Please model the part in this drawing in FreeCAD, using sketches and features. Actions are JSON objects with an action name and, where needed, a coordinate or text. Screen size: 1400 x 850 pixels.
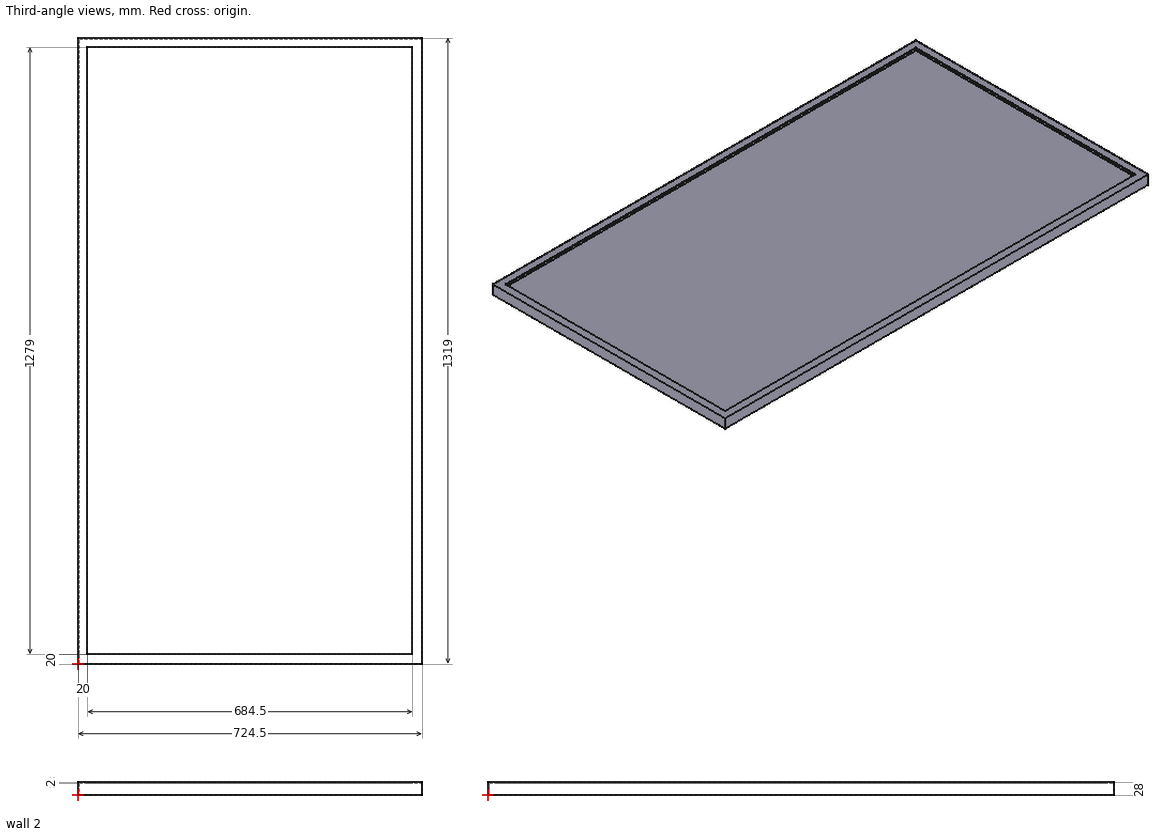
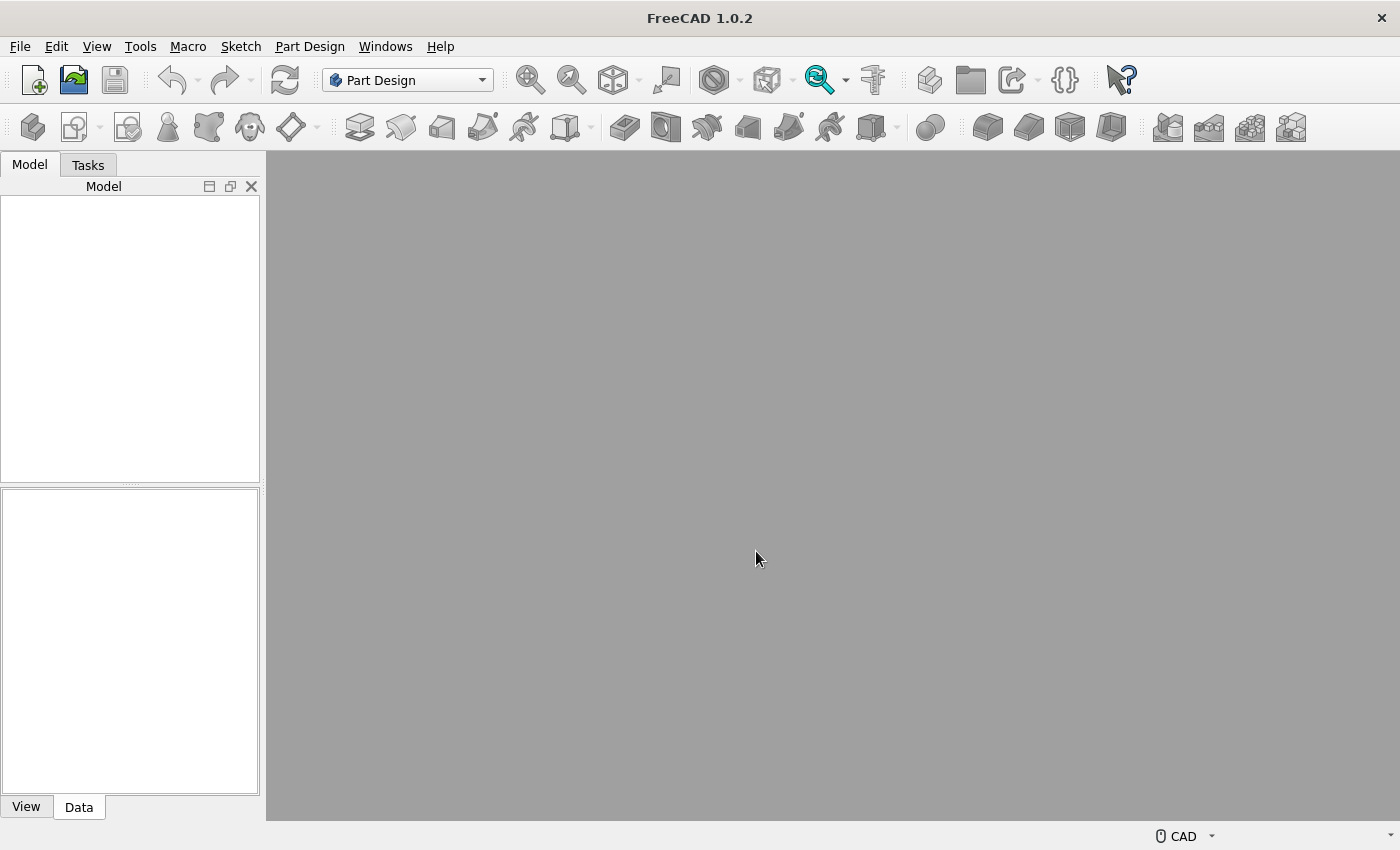
{"action": "left_click", "coordinate": [33, 80]}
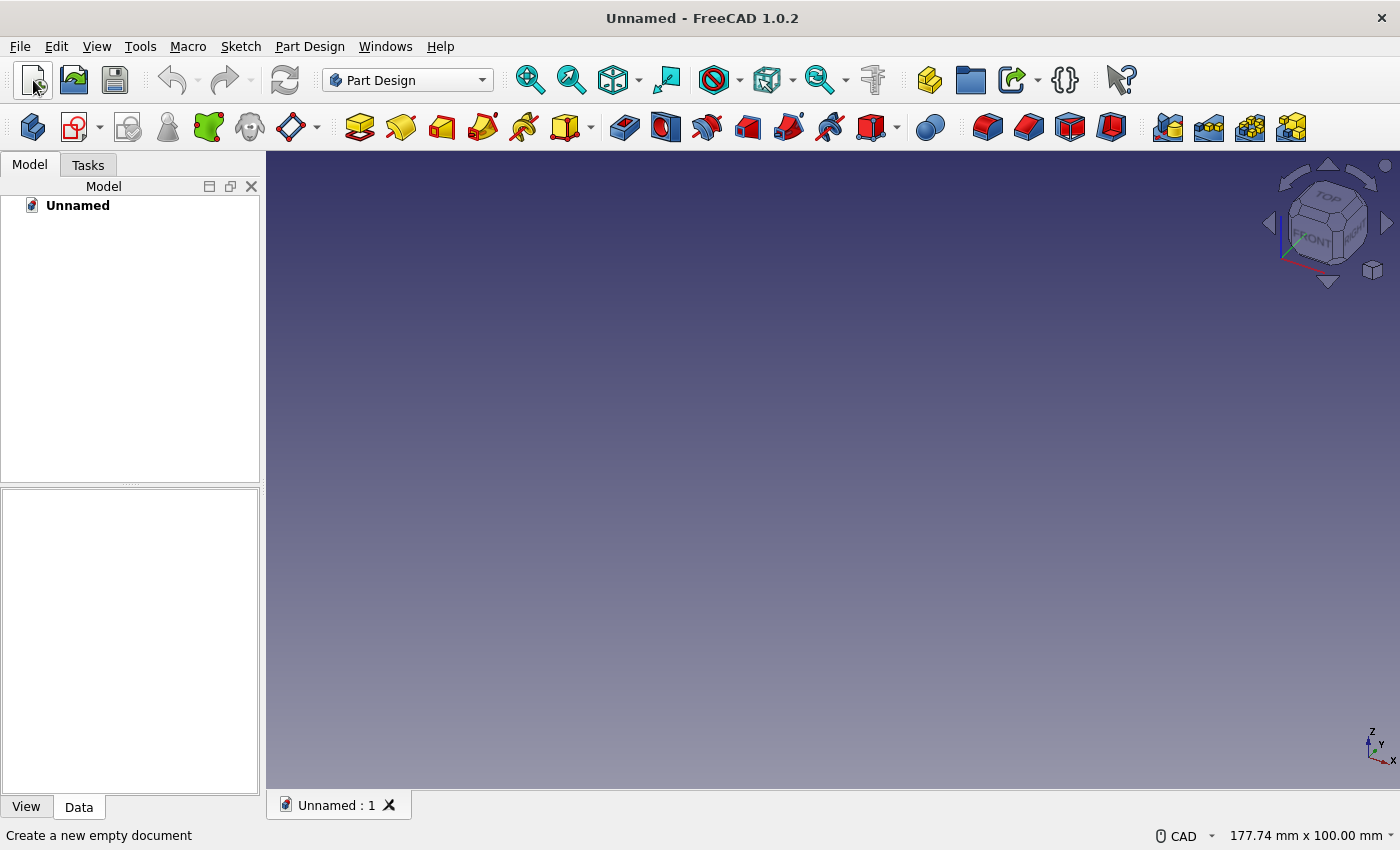
{"action": "left_click", "coordinate": [74, 128]}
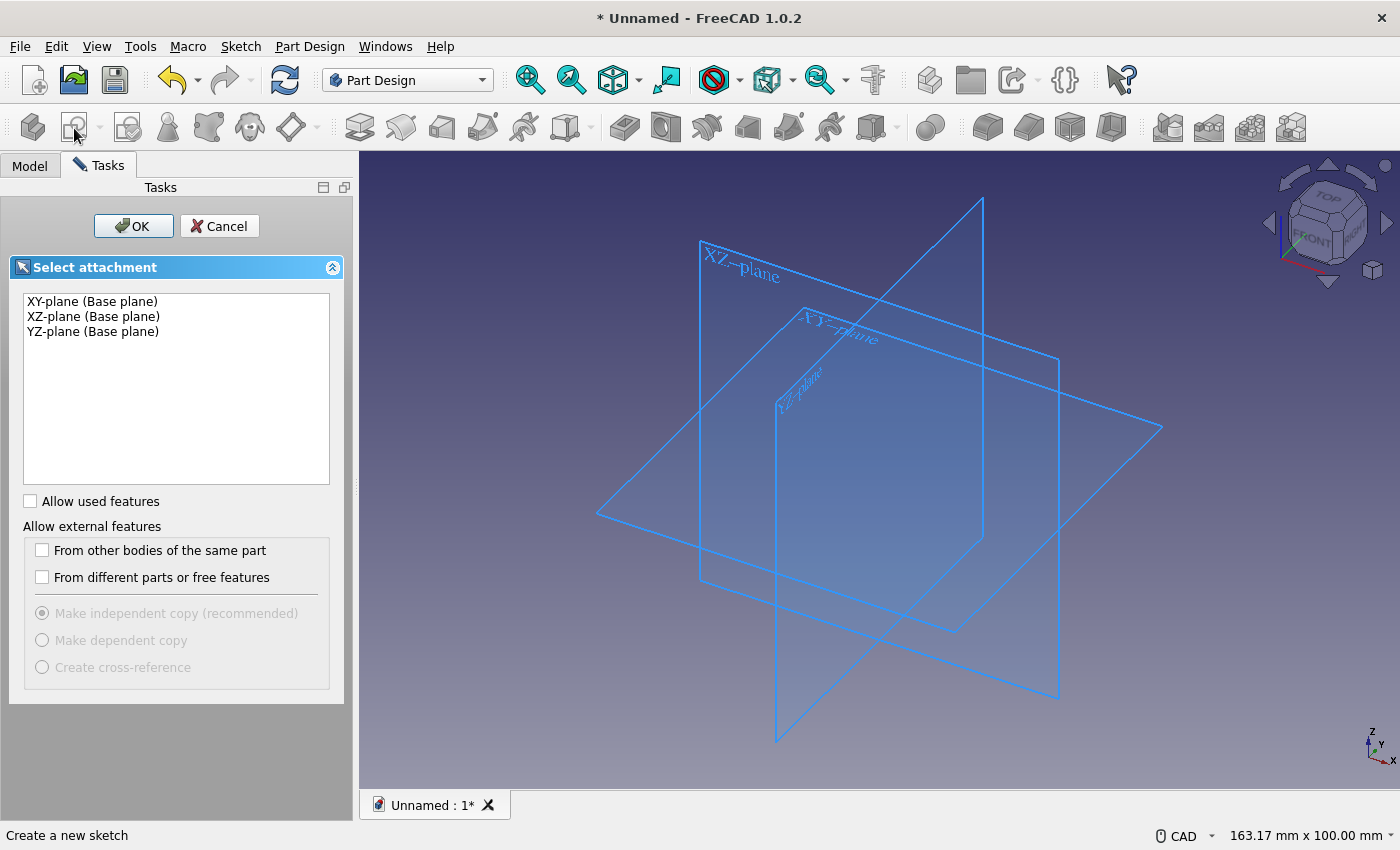
{"action": "left_click", "coordinate": [84, 302]}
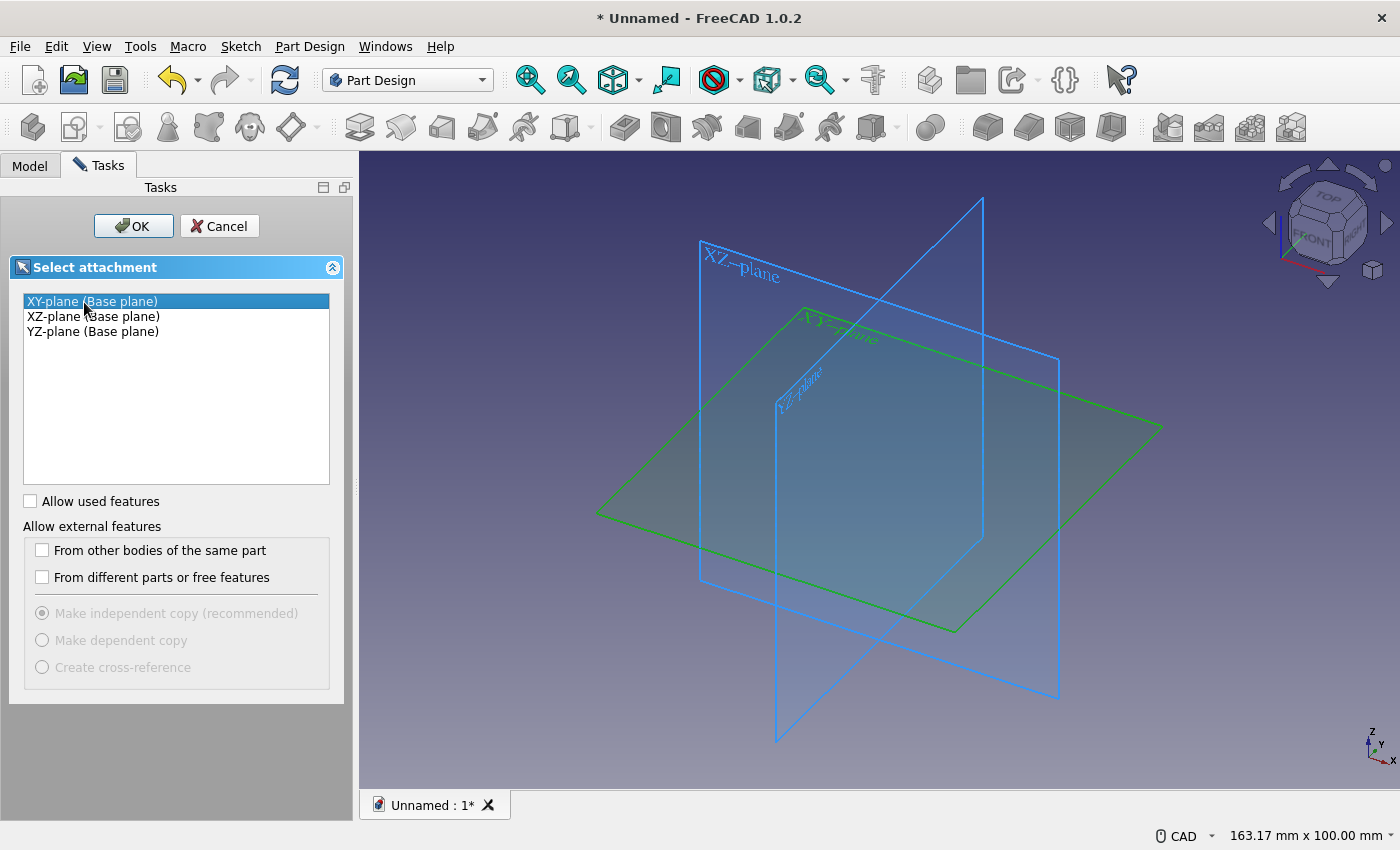
{"action": "left_click", "coordinate": [134, 226]}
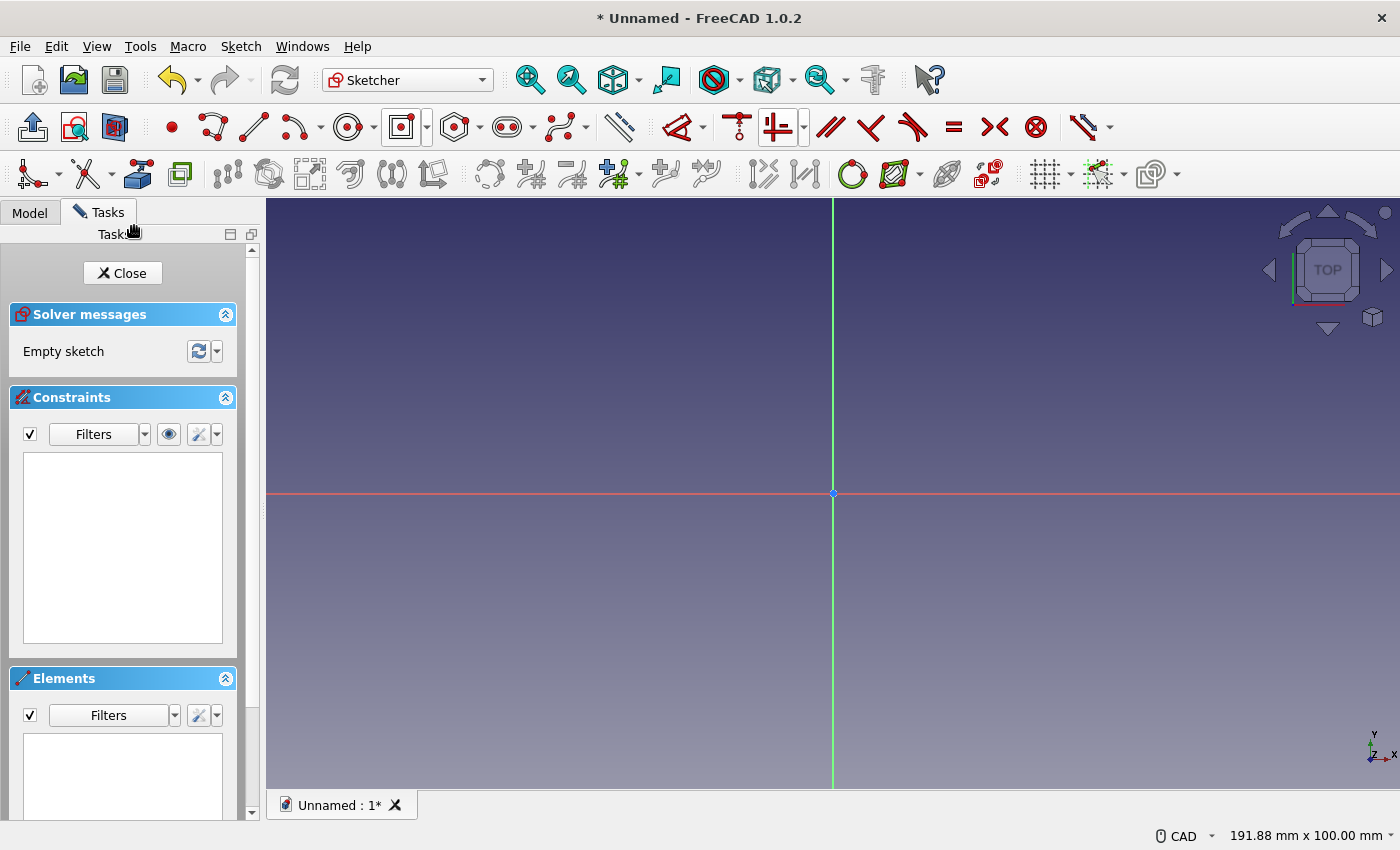
{"action": "scroll", "coordinate": [649, 698], "scroll_direction": "down", "scroll_amount": 15}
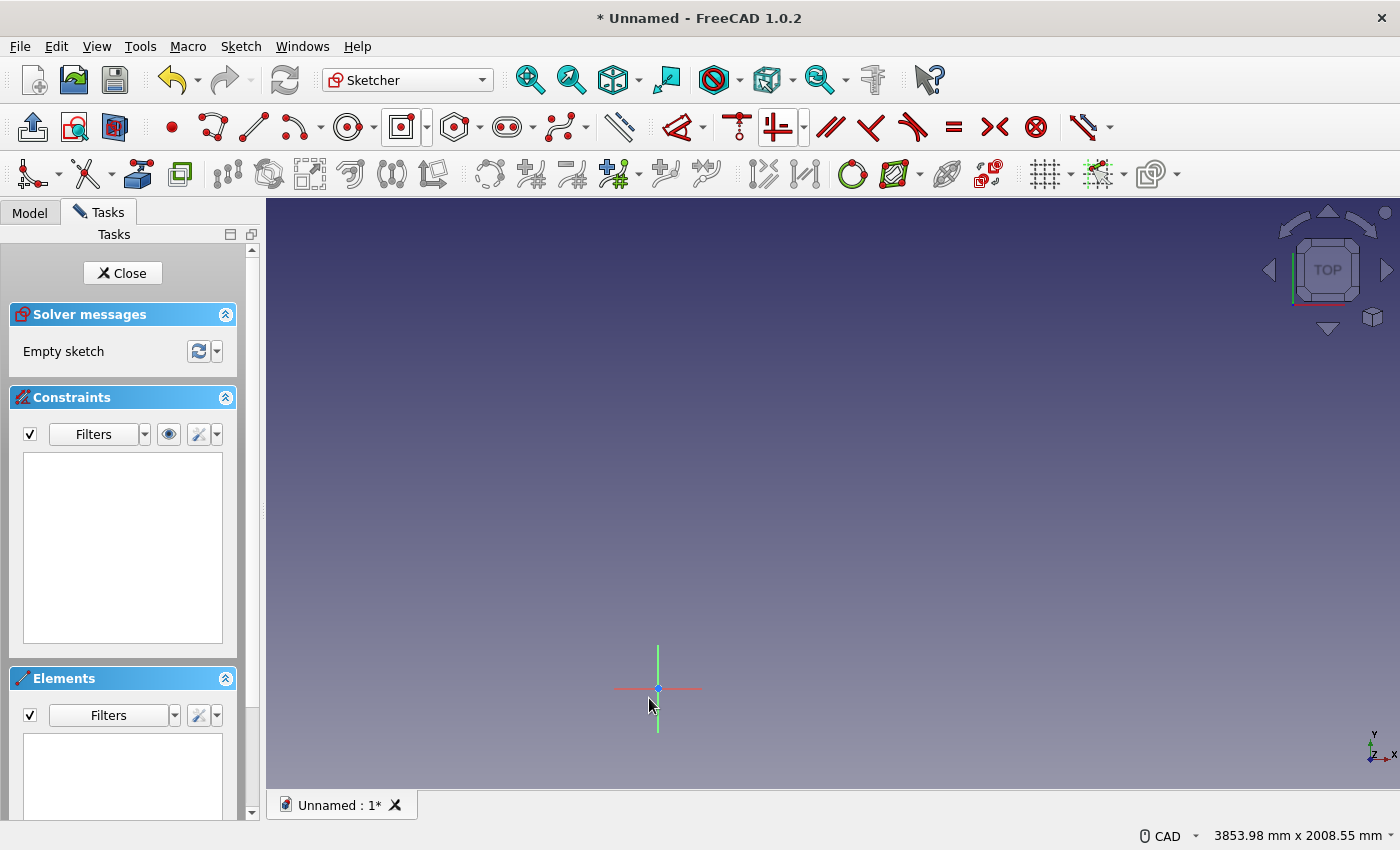
{"action": "left_click", "coordinate": [426, 128]}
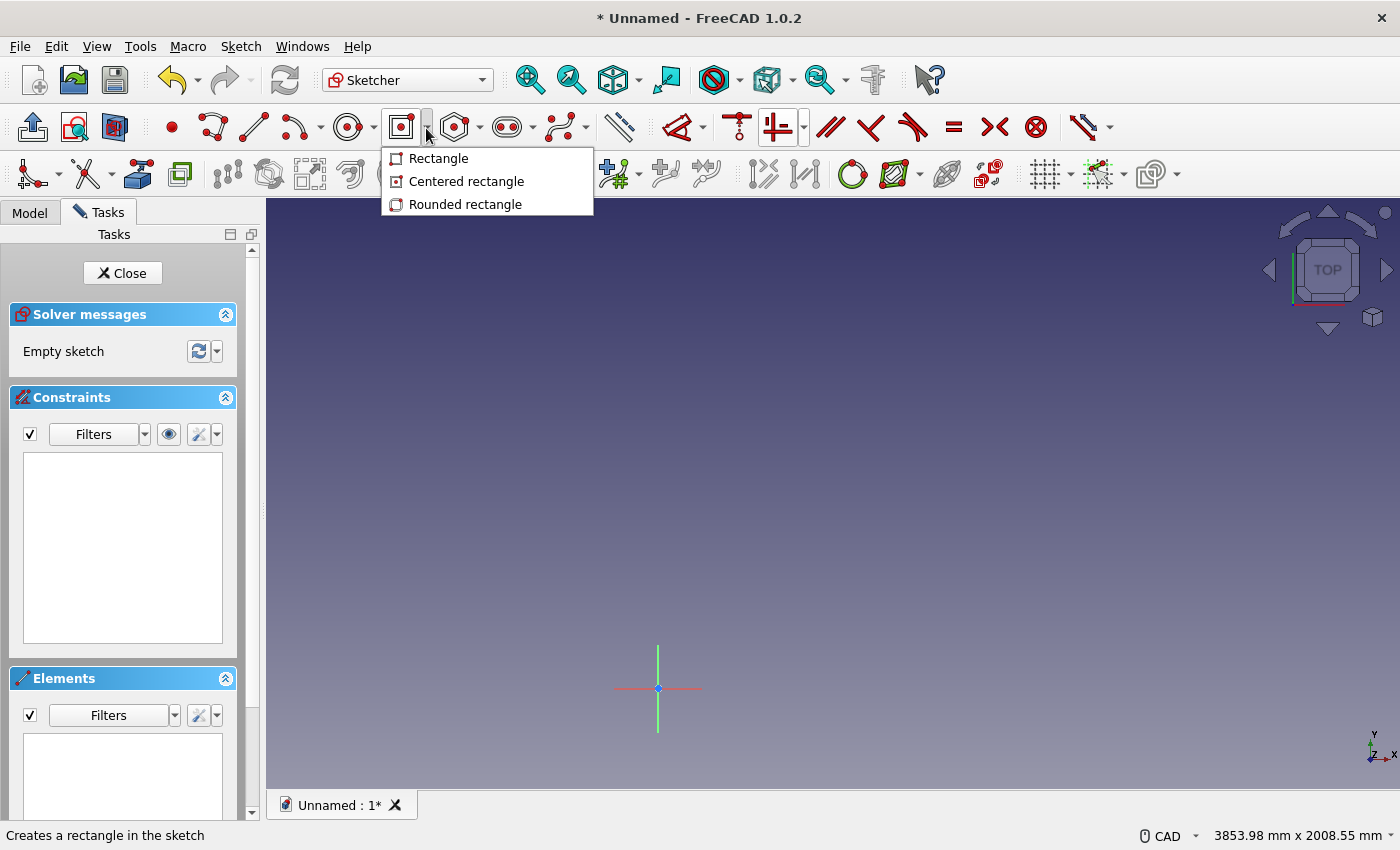
{"action": "left_click", "coordinate": [488, 158]}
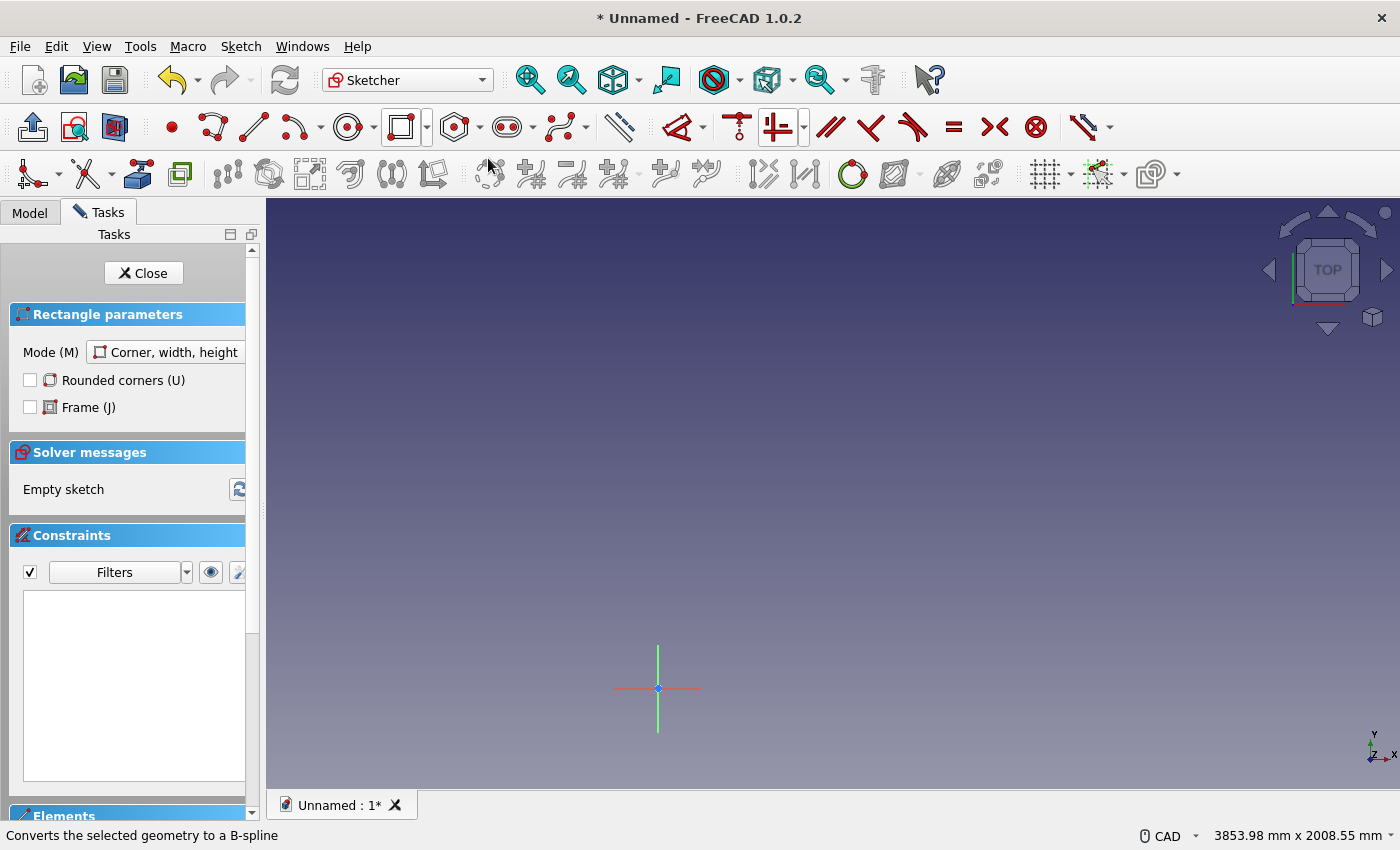
{"action": "left_click", "coordinate": [658, 689]}
{"action": "mouse_move", "coordinate": [872, 301]}